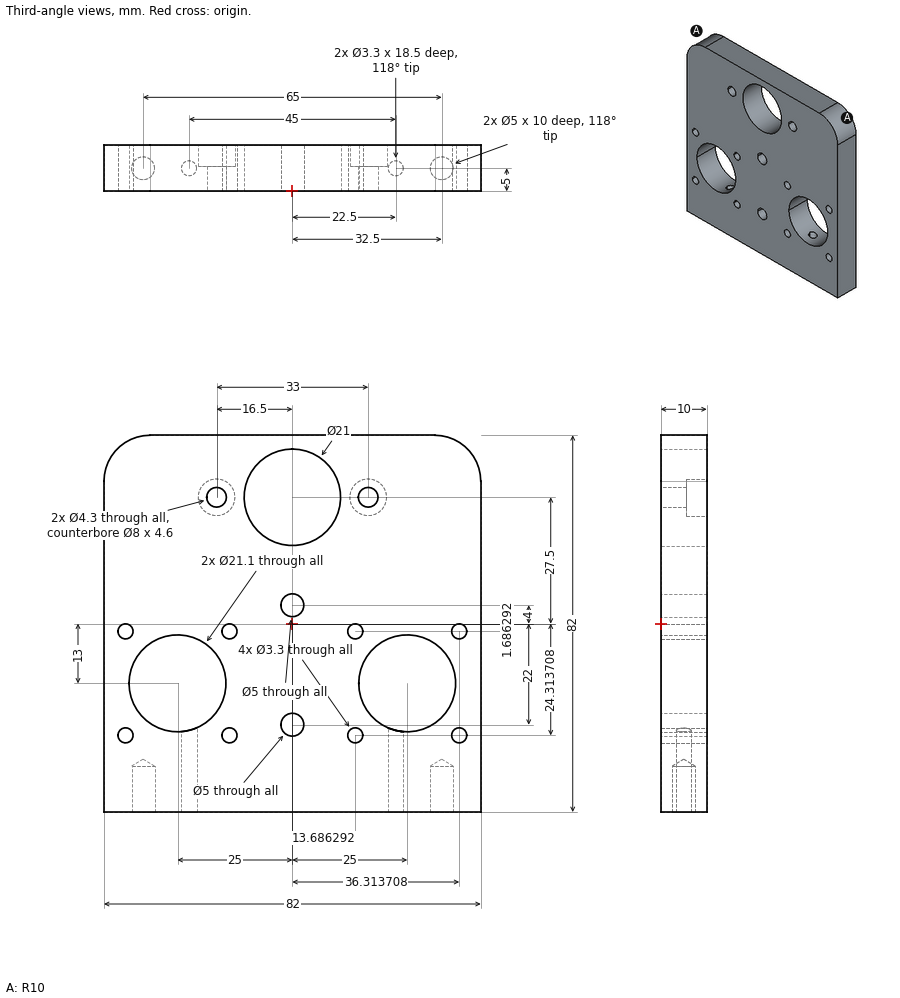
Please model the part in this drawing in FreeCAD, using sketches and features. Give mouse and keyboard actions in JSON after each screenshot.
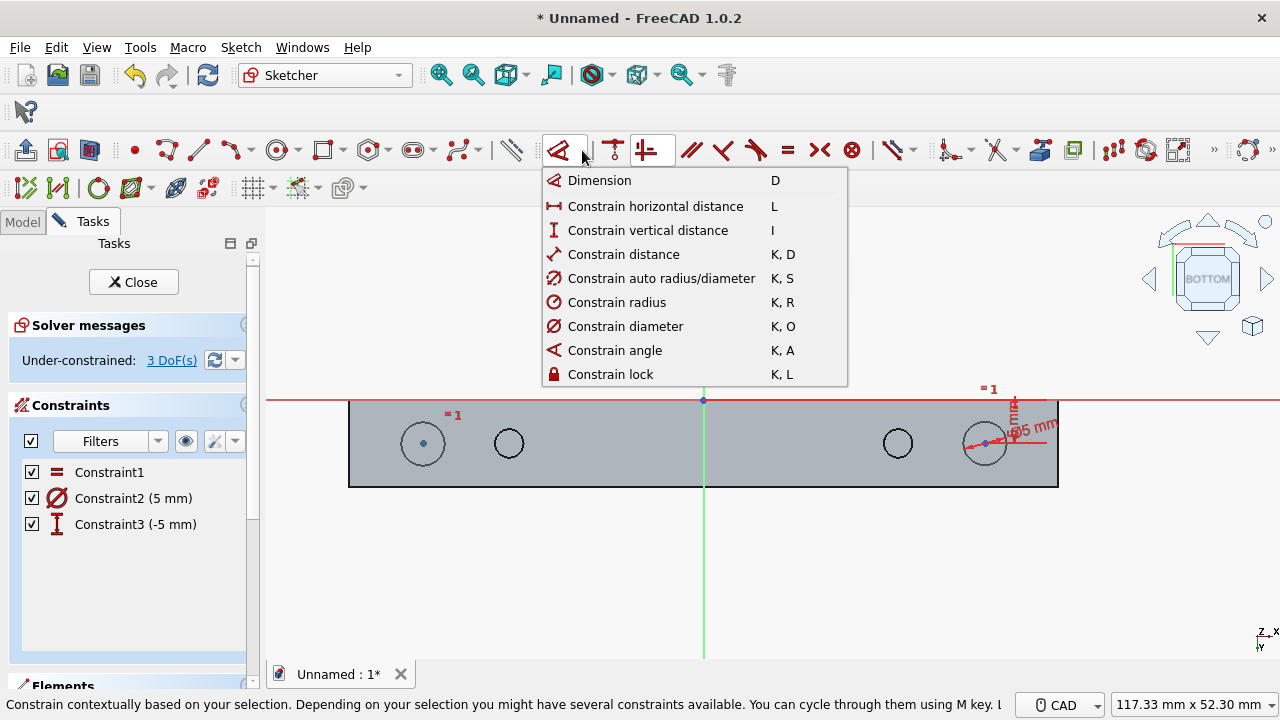
{"action": "left_click", "coordinate": [695, 230]}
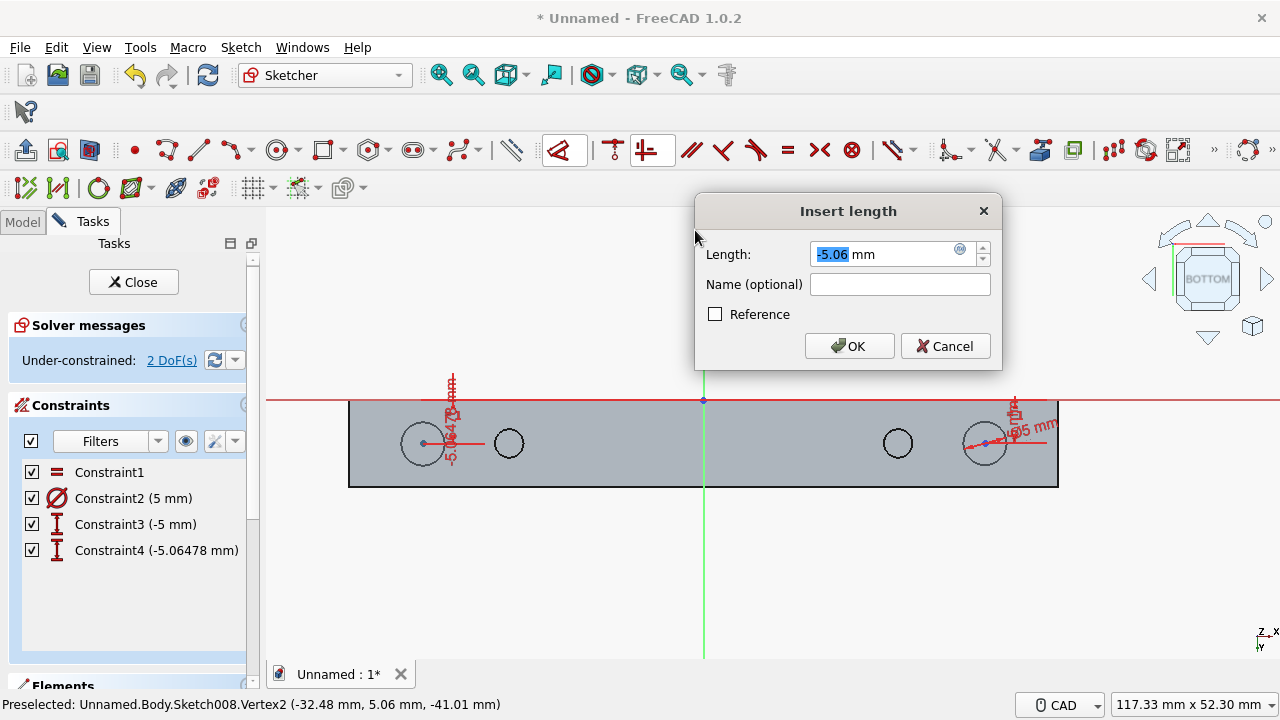
{"action": "type", "text": "-5"}
{"action": "key", "text": "Return"}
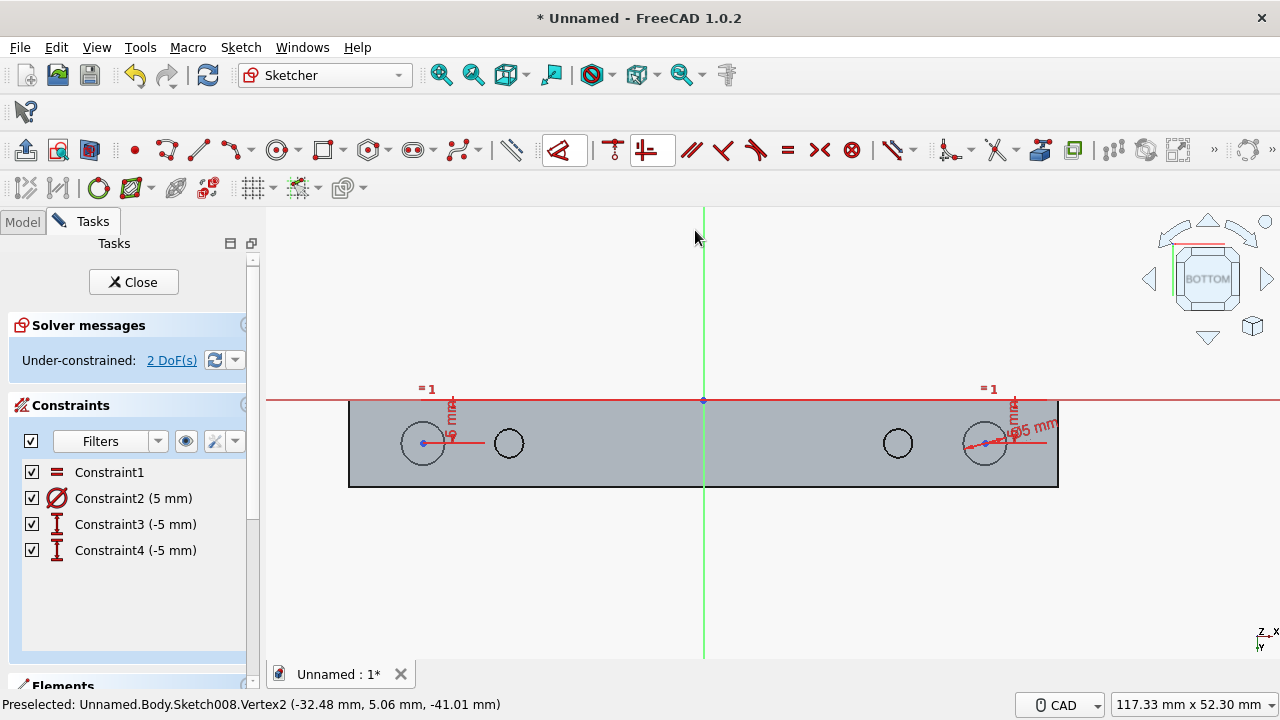
{"action": "left_click", "coordinate": [985, 443]}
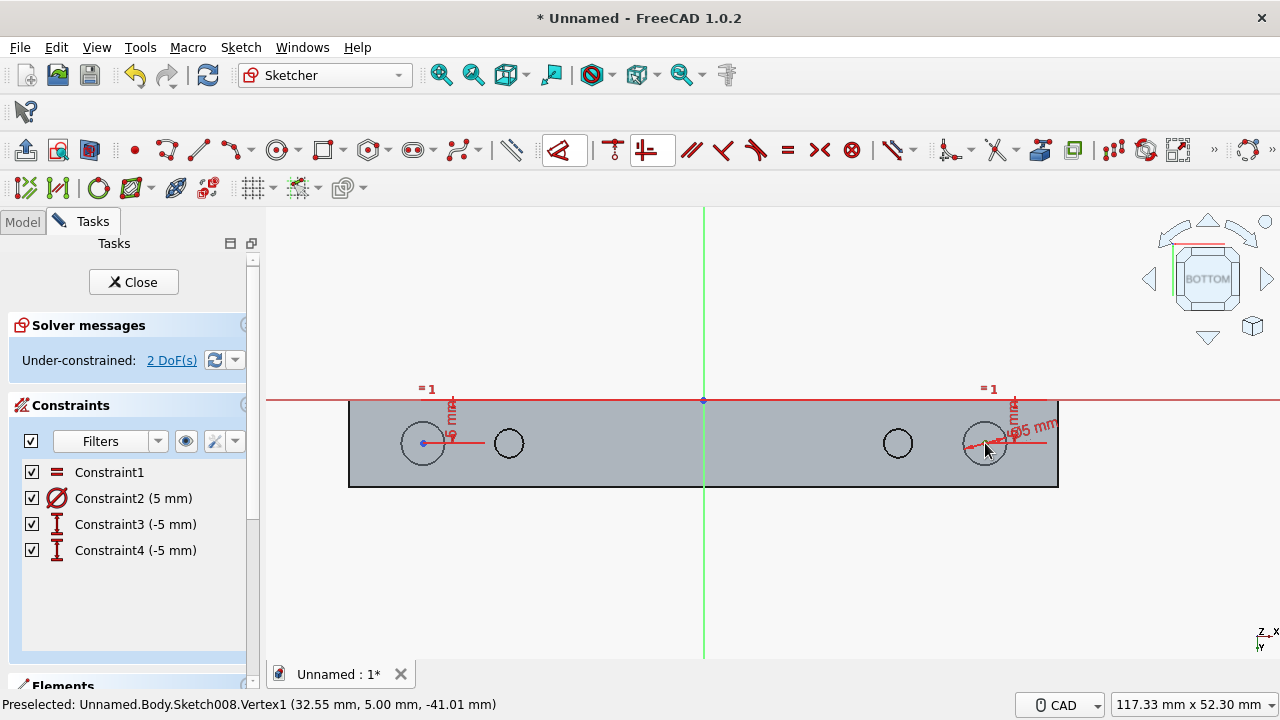
{"action": "left_click", "coordinate": [423, 443]}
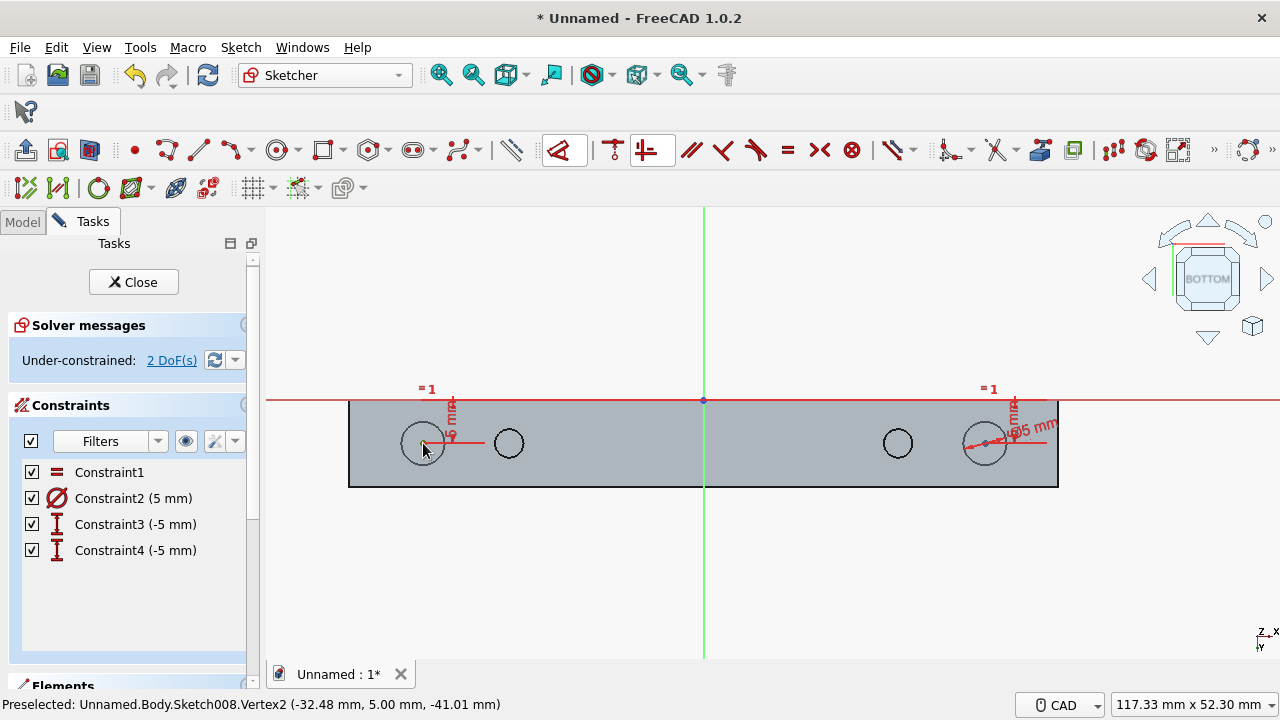
{"action": "key", "text": "l"}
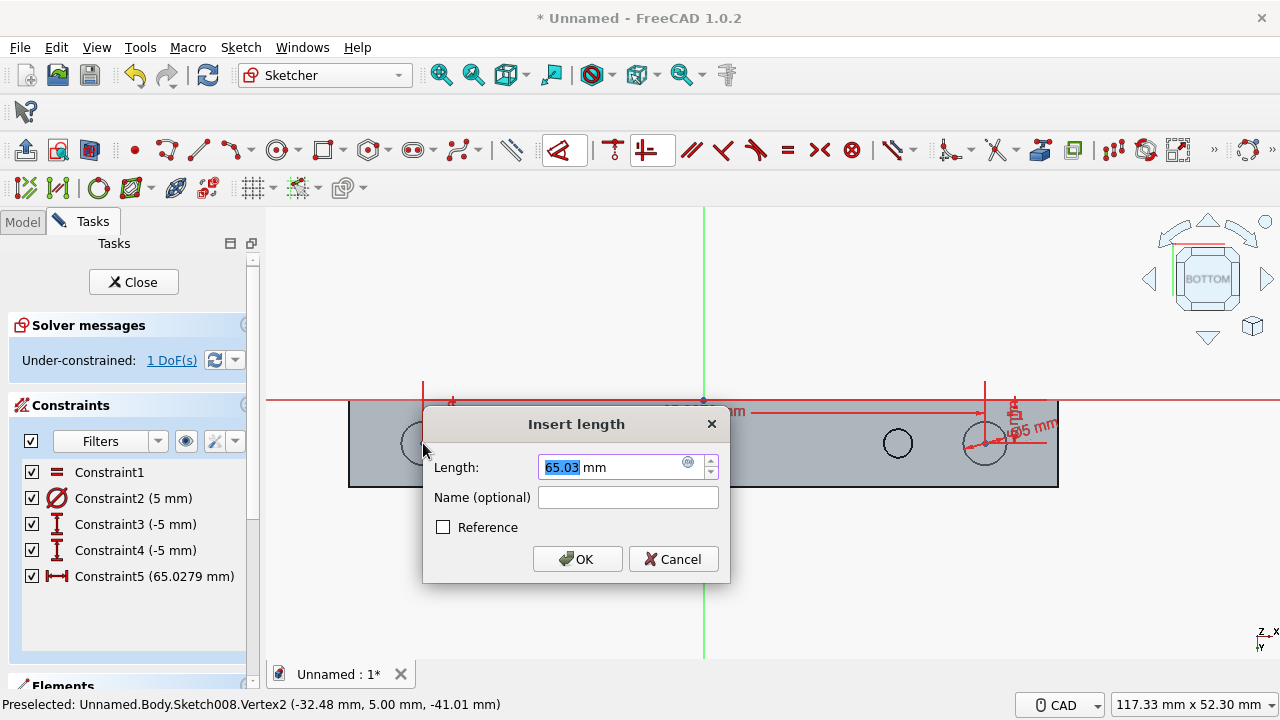
{"action": "type", "text": "65"}
{"action": "key", "text": "Return"}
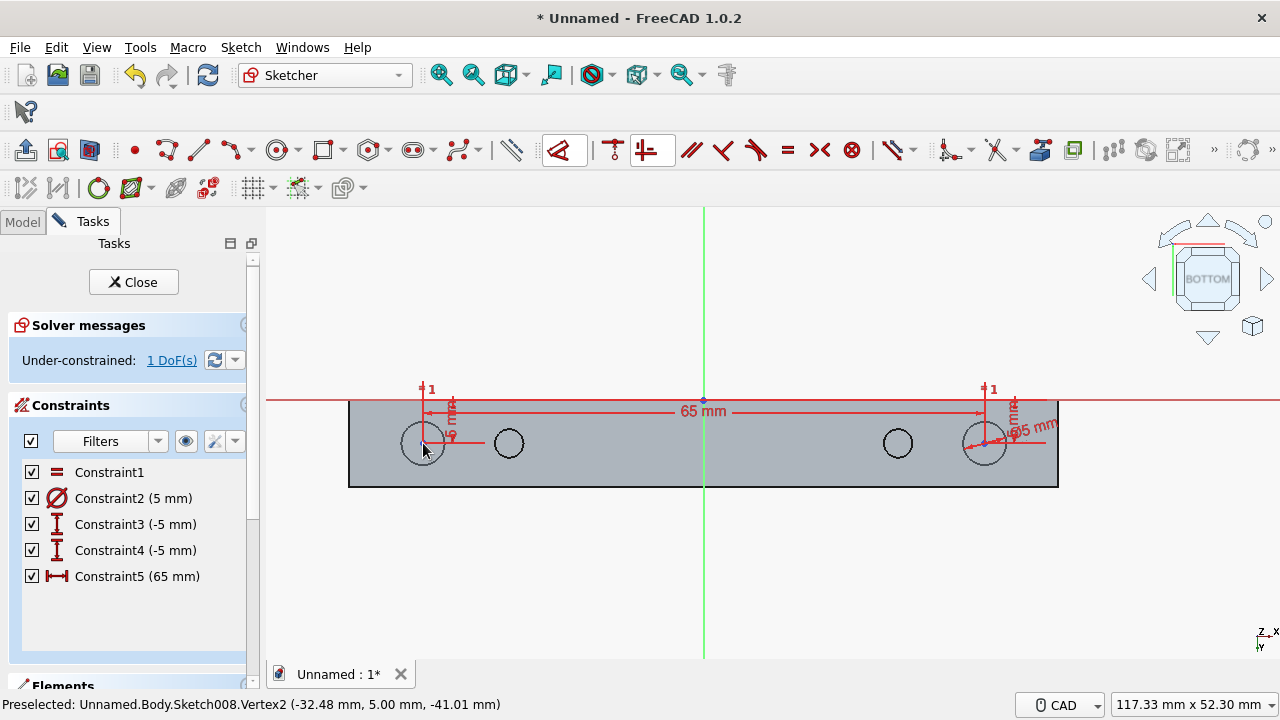
{"action": "left_click", "coordinate": [985, 443]}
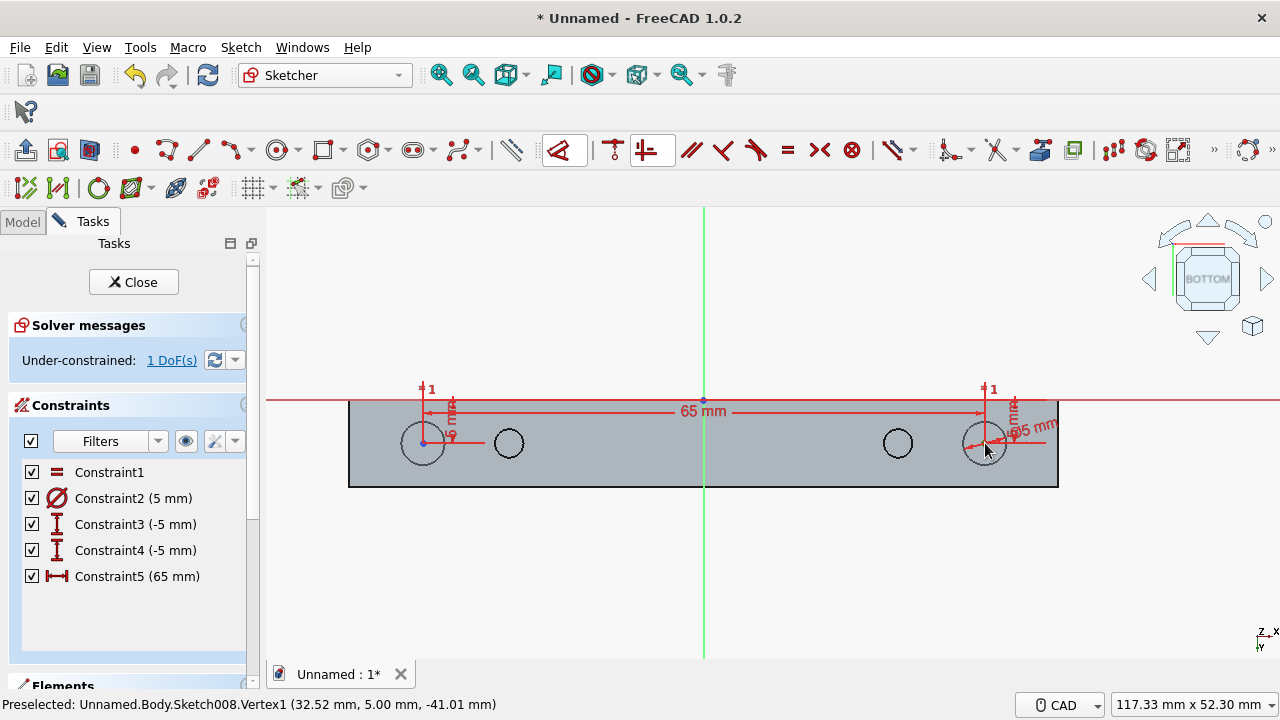
{"action": "key", "text": "l"}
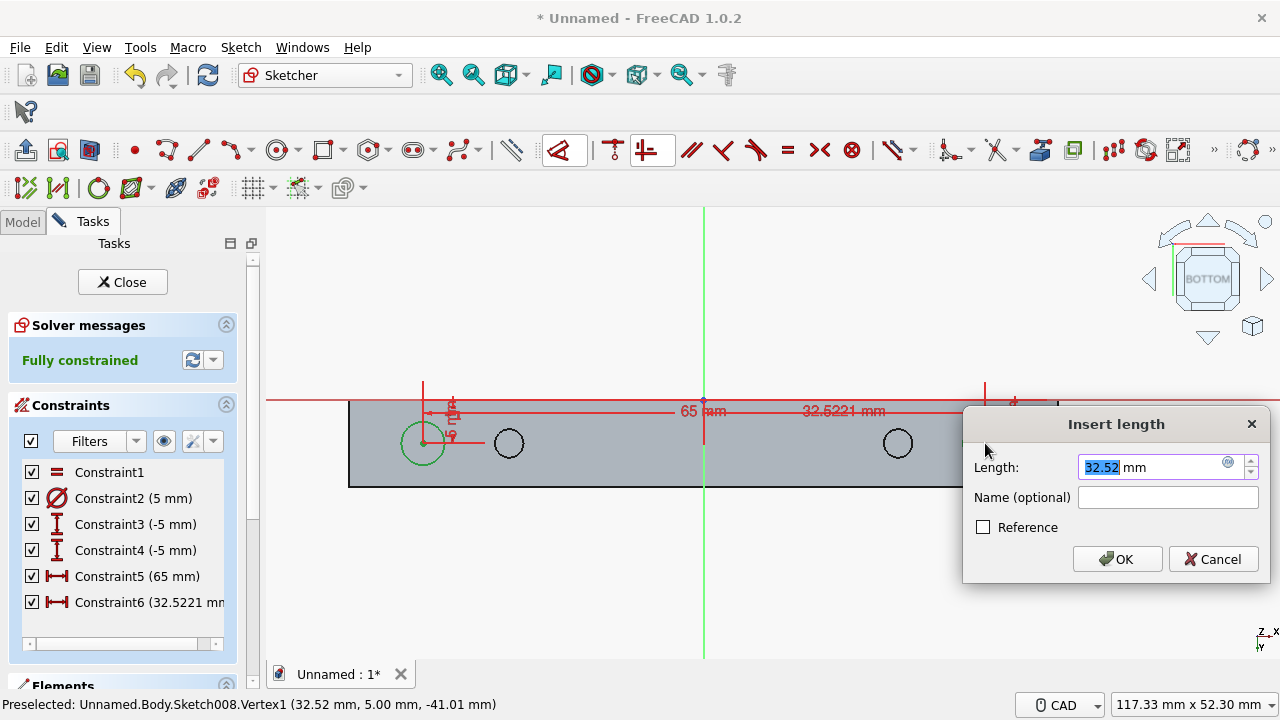
{"action": "type", "text": "32.5"}
{"action": "key", "text": "Return"}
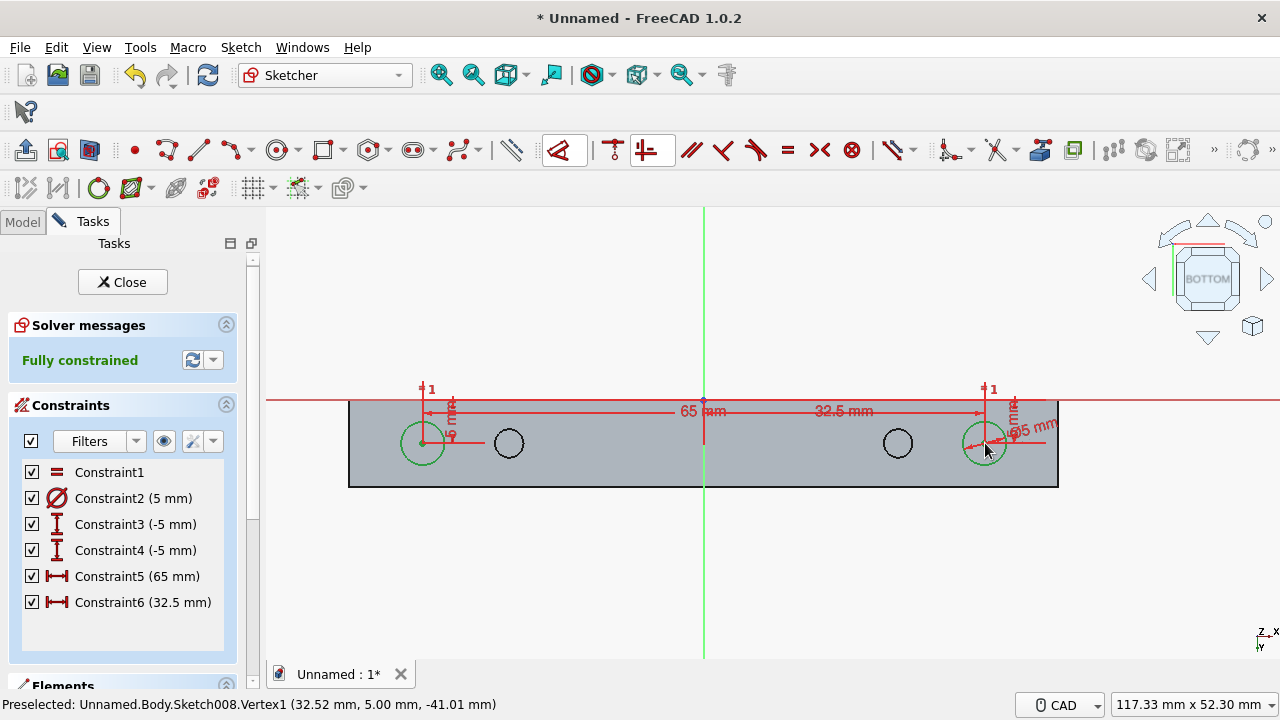
{"action": "left_click", "coordinate": [123, 282]}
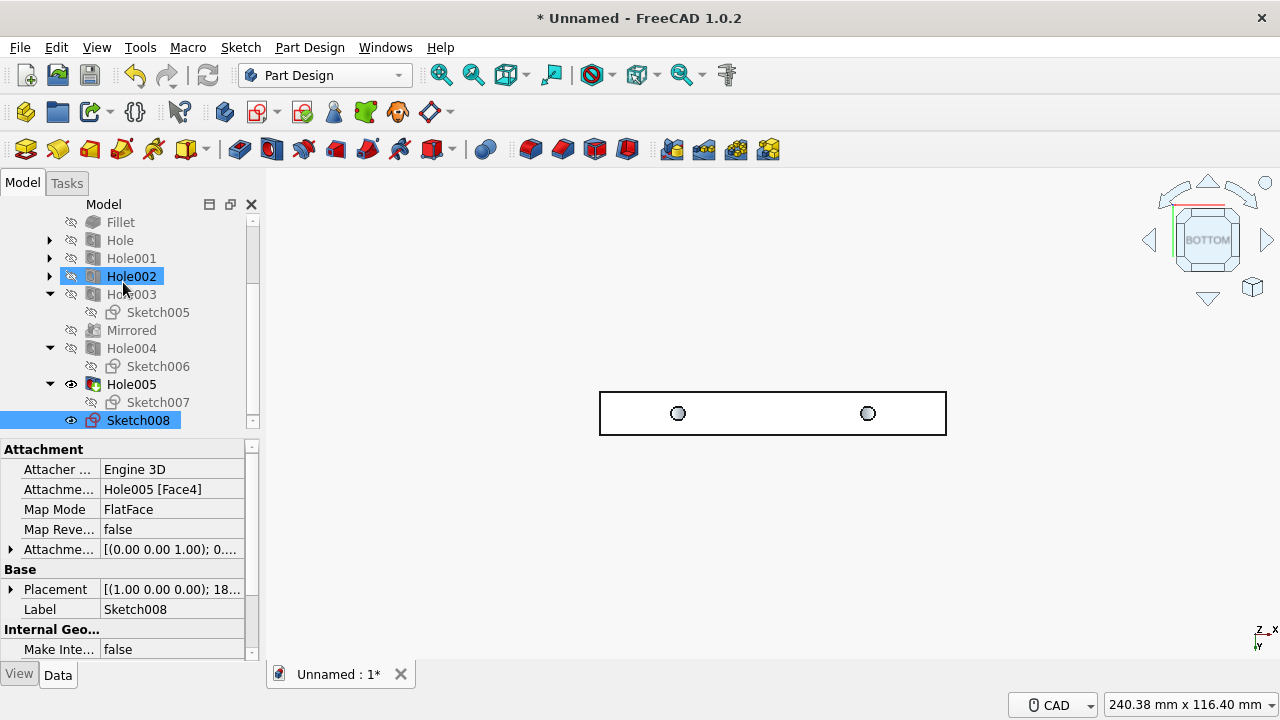
{"action": "left_click", "coordinate": [272, 150]}